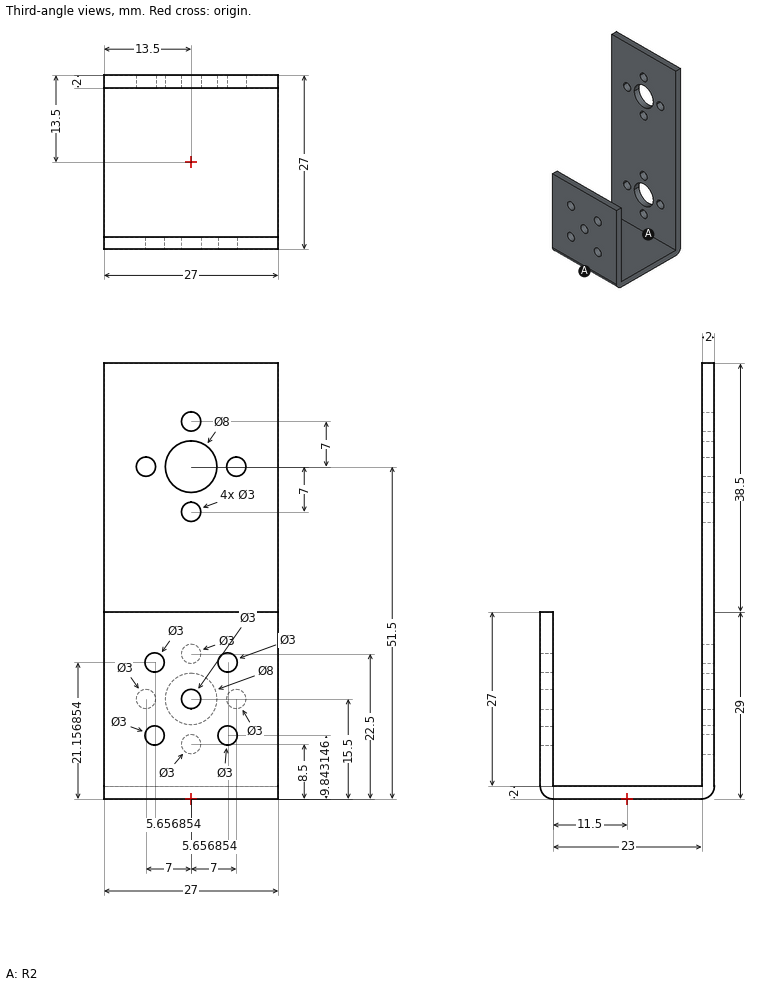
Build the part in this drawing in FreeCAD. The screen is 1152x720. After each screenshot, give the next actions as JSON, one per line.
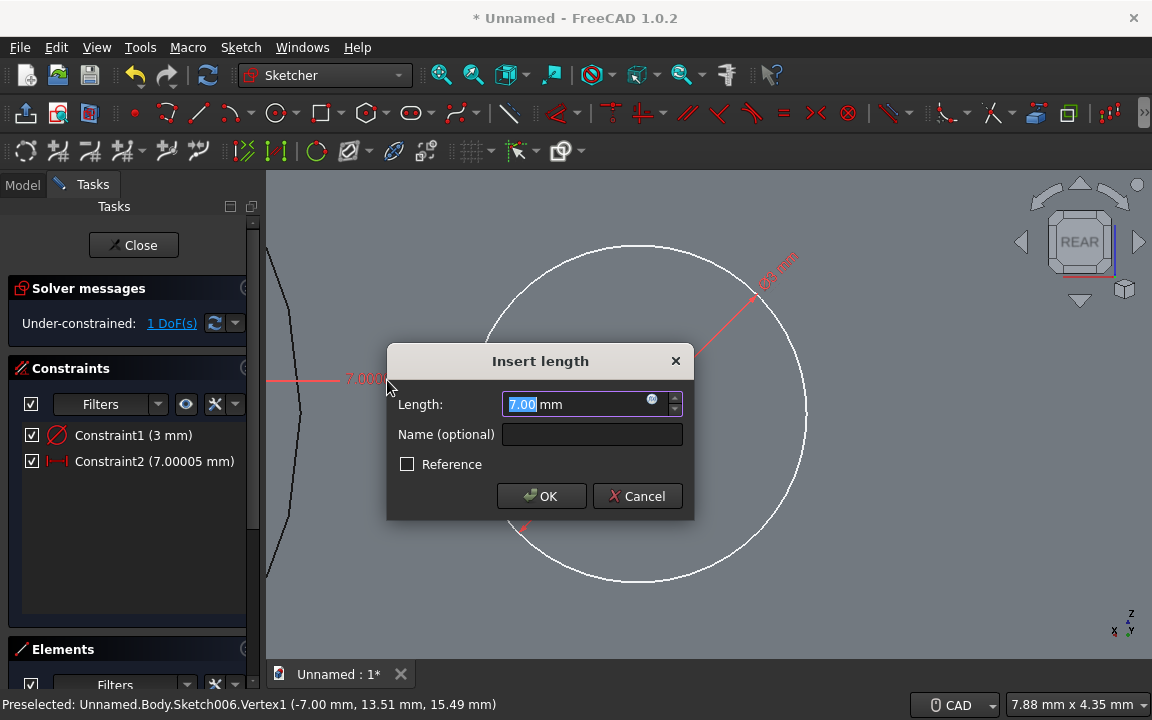
{"action": "type", "text": "7"}
{"action": "key", "text": "Return"}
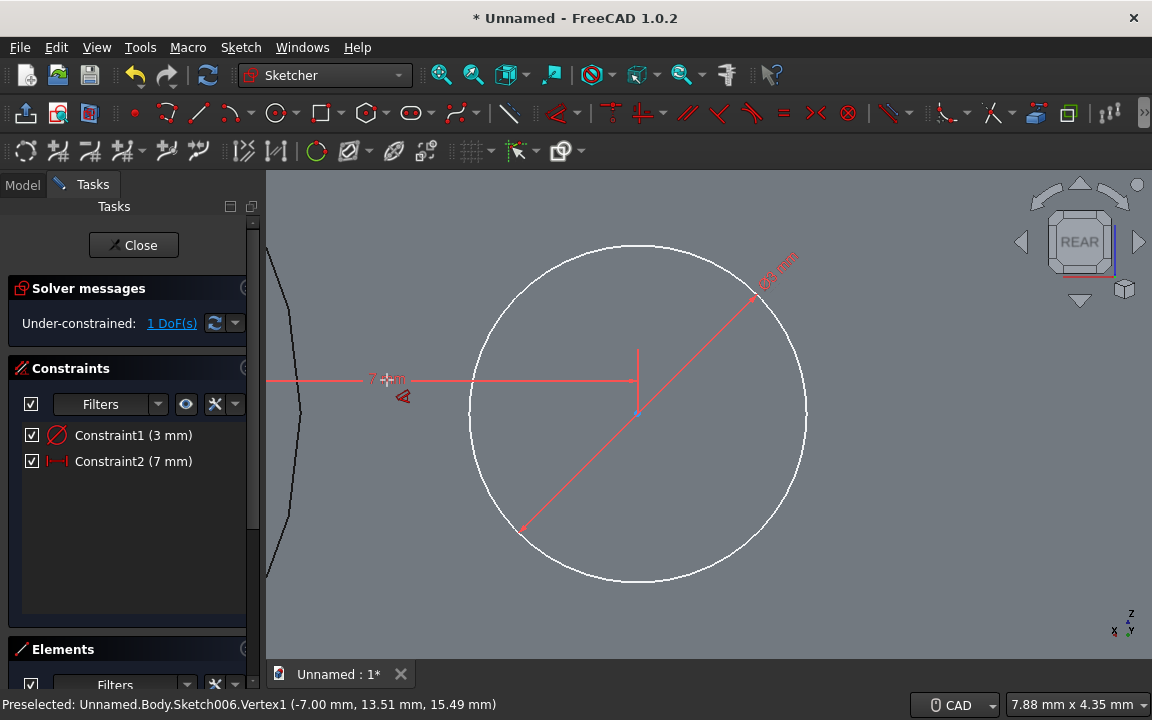
{"action": "left_click", "coordinate": [638, 414]}
{"action": "left_click", "coordinate": [672, 522]}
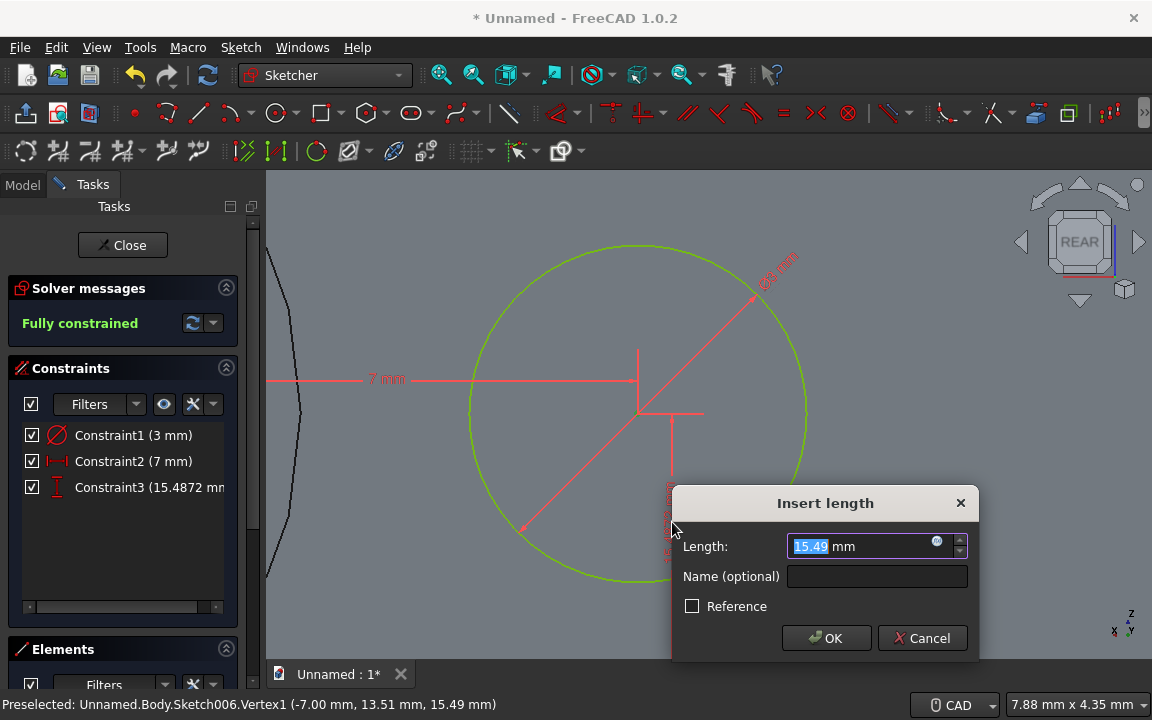
{"action": "type", "text": "15.5"}
{"action": "key", "text": "Return"}
{"action": "key", "text": "Escape"}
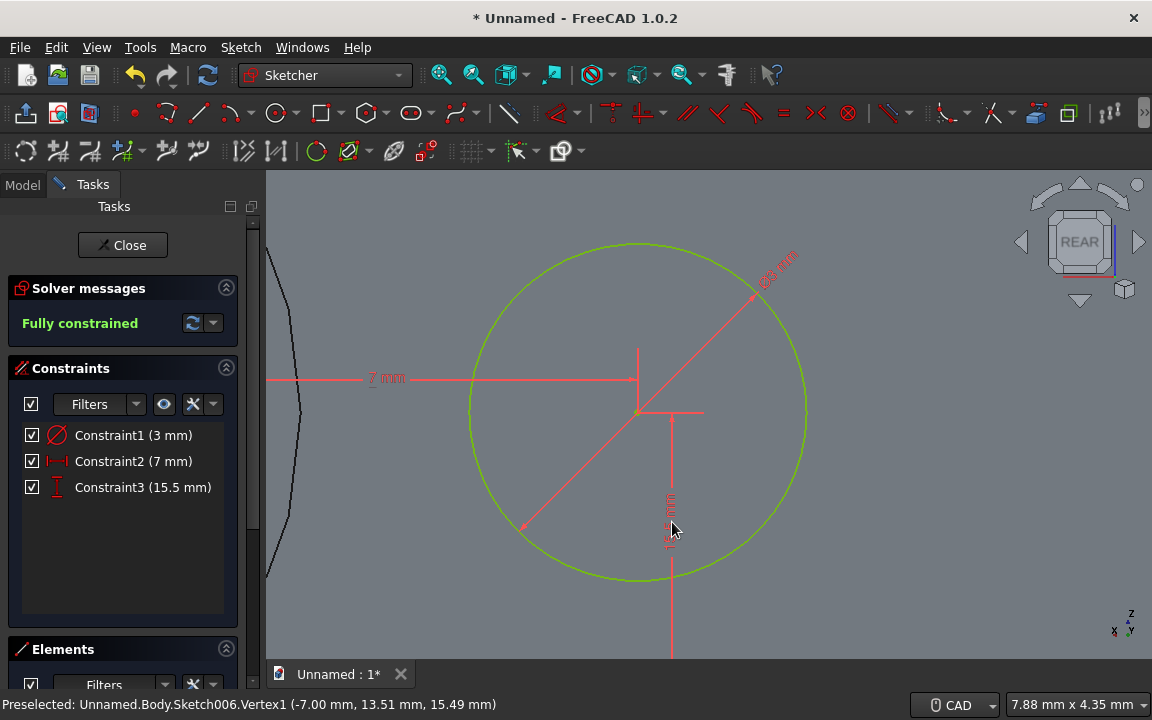
{"action": "left_click", "coordinate": [123, 245]}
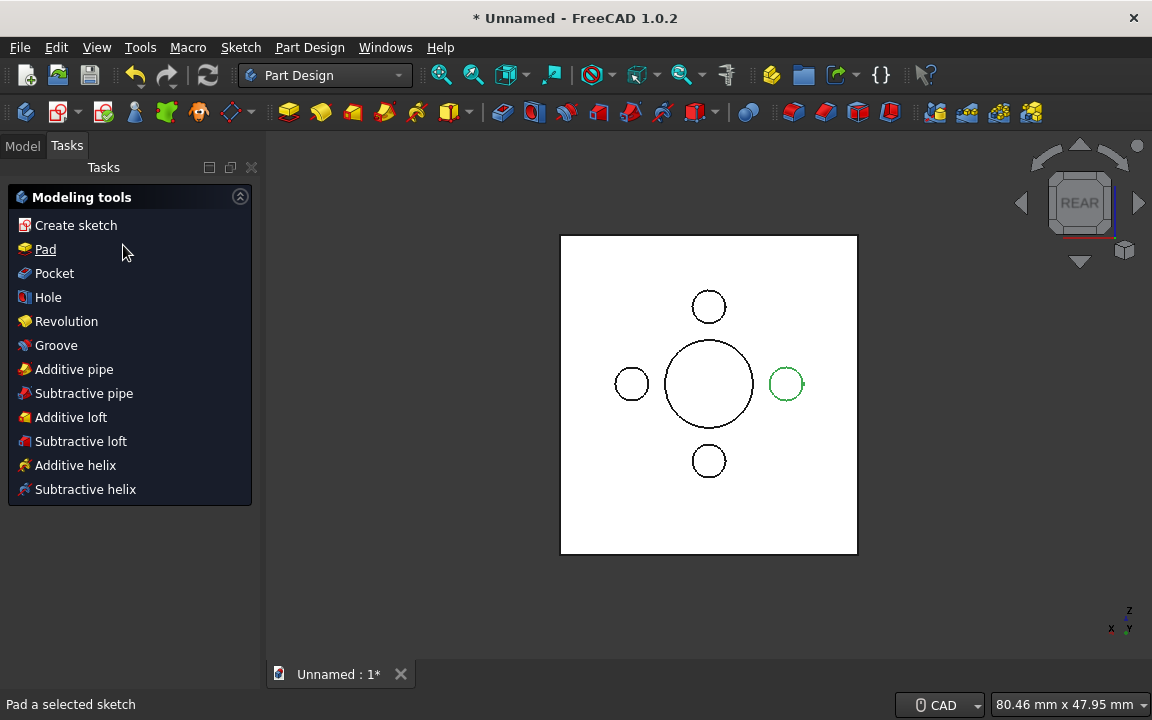
{"action": "left_click", "coordinate": [504, 112]}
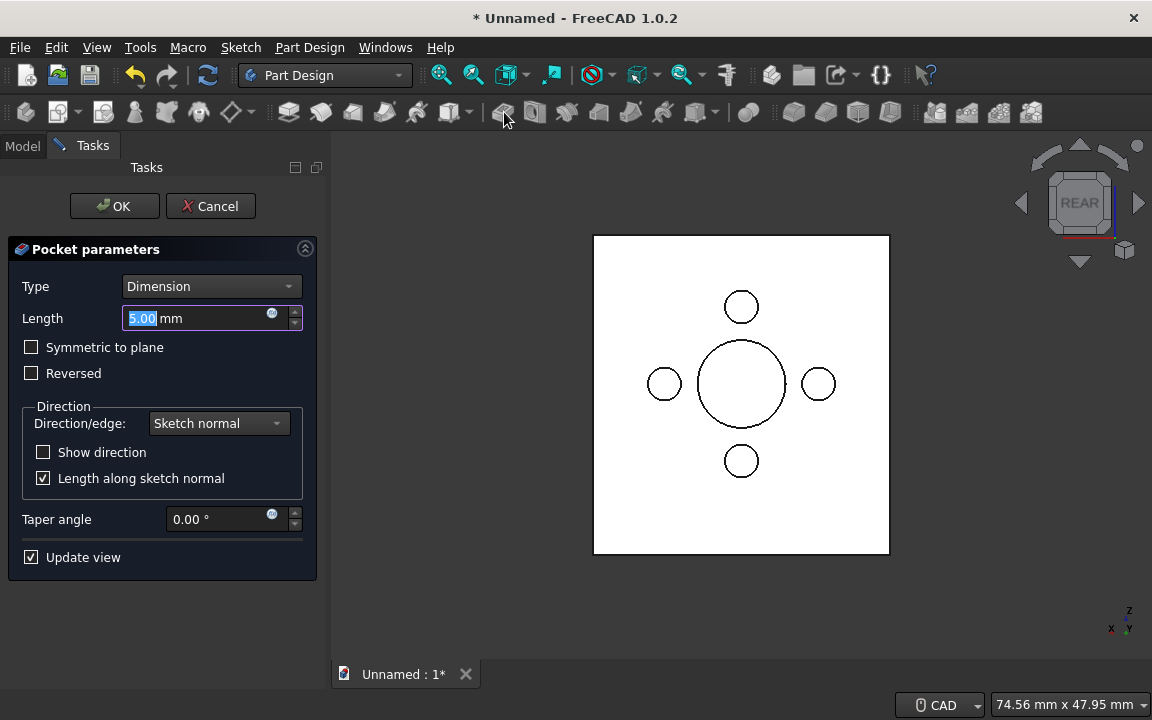
{"action": "left_click", "coordinate": [212, 286]}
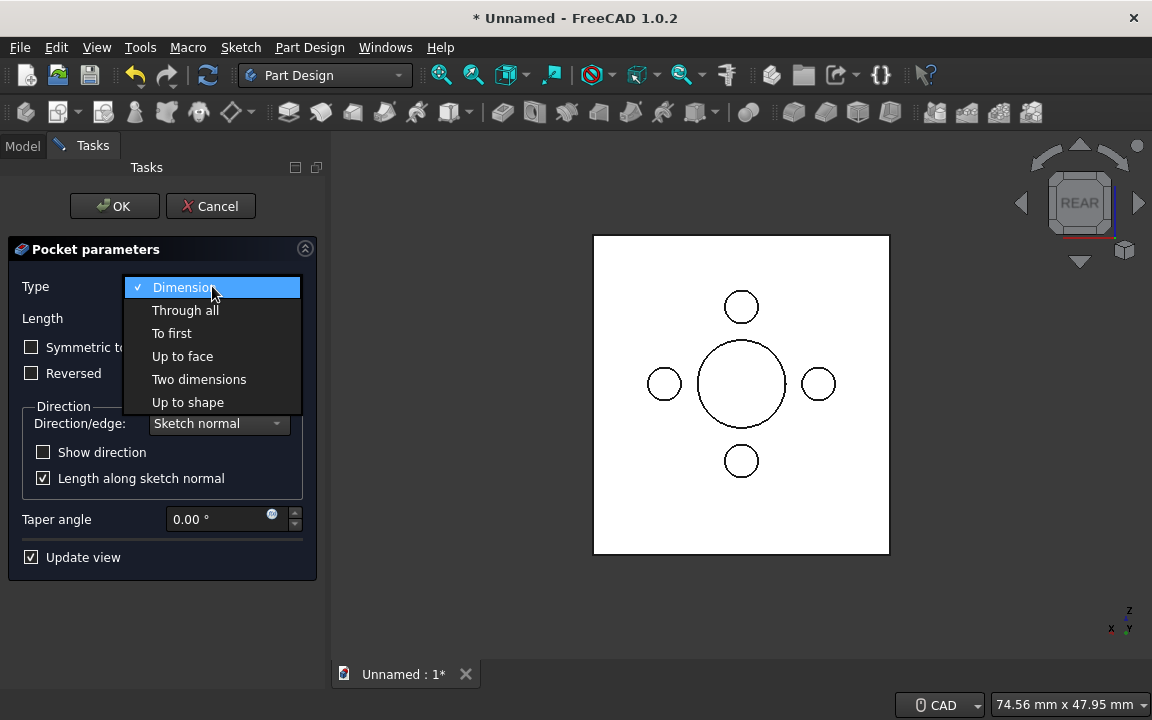
{"action": "left_click", "coordinate": [212, 334]}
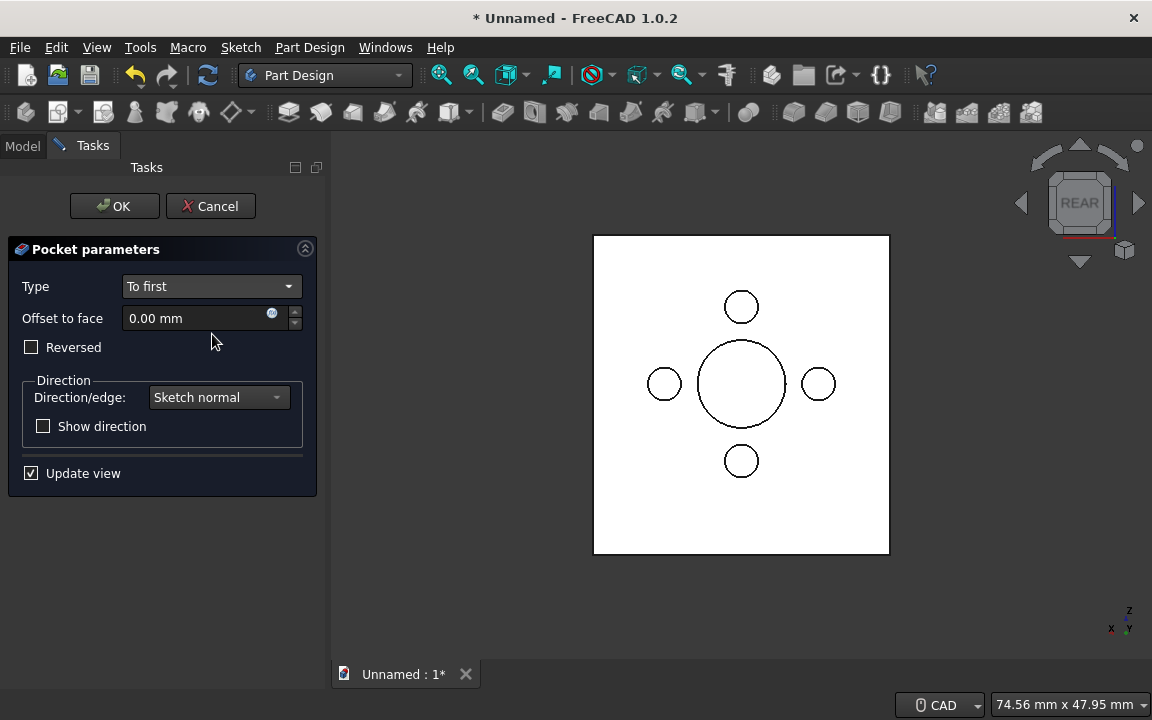
{"action": "left_click", "coordinate": [115, 206]}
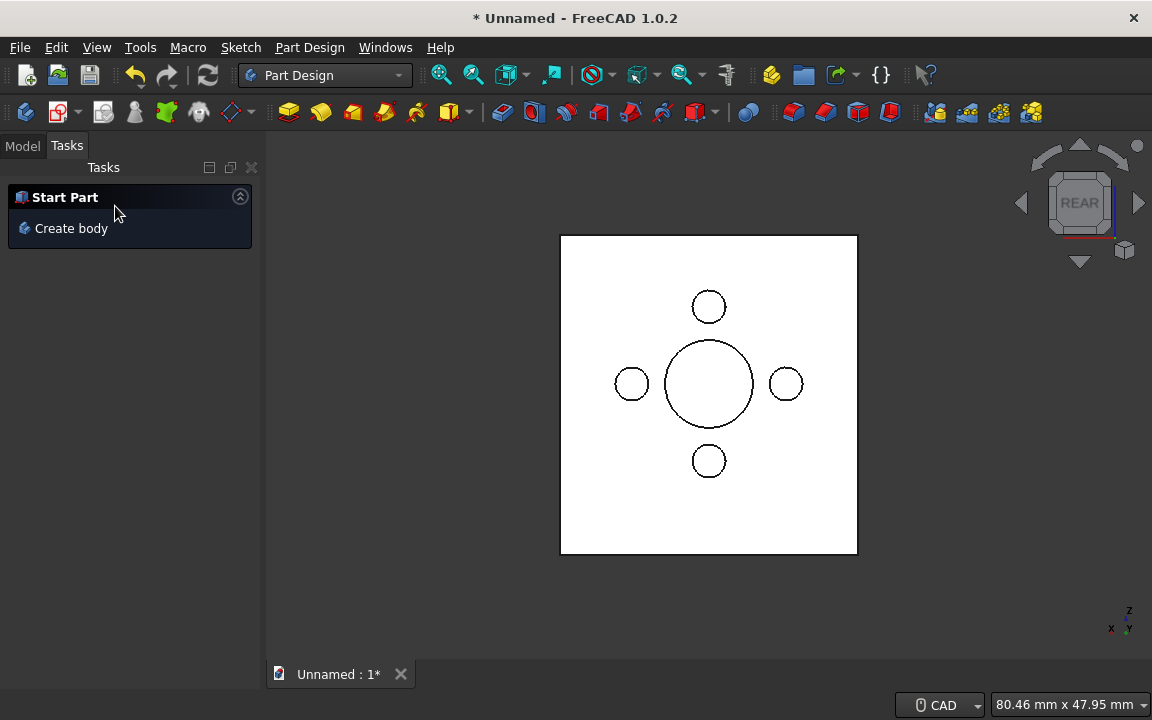
{"action": "key", "text": "0"}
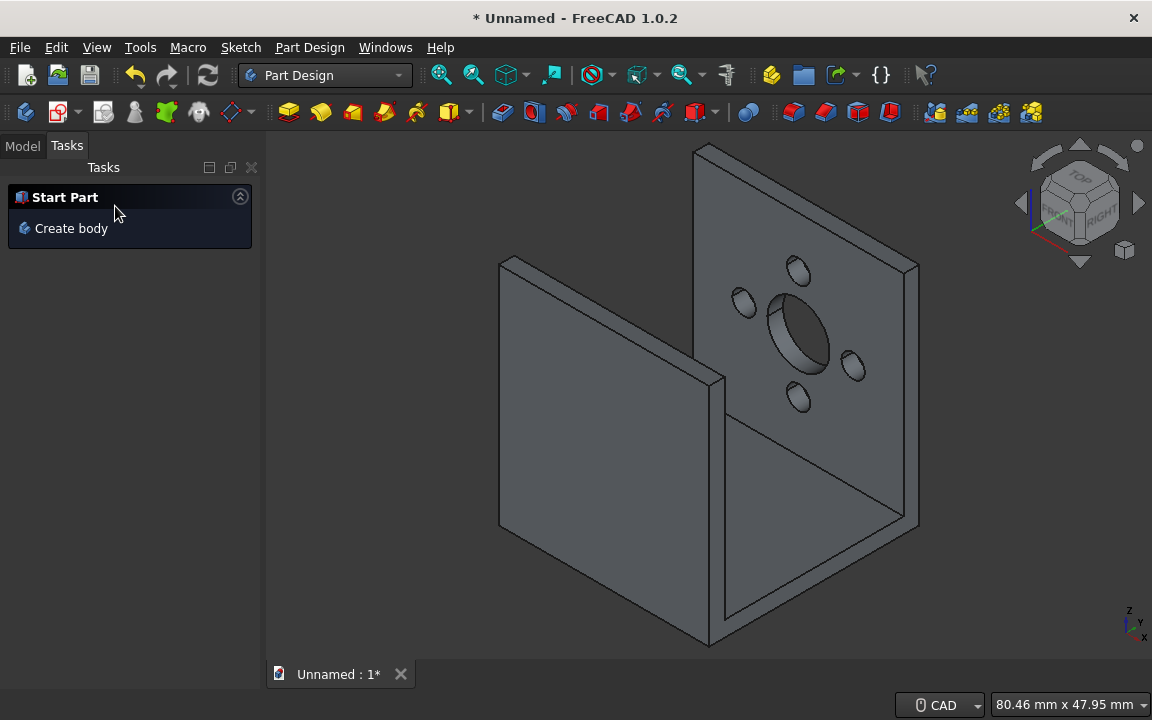
{"action": "left_click", "coordinate": [604, 455]}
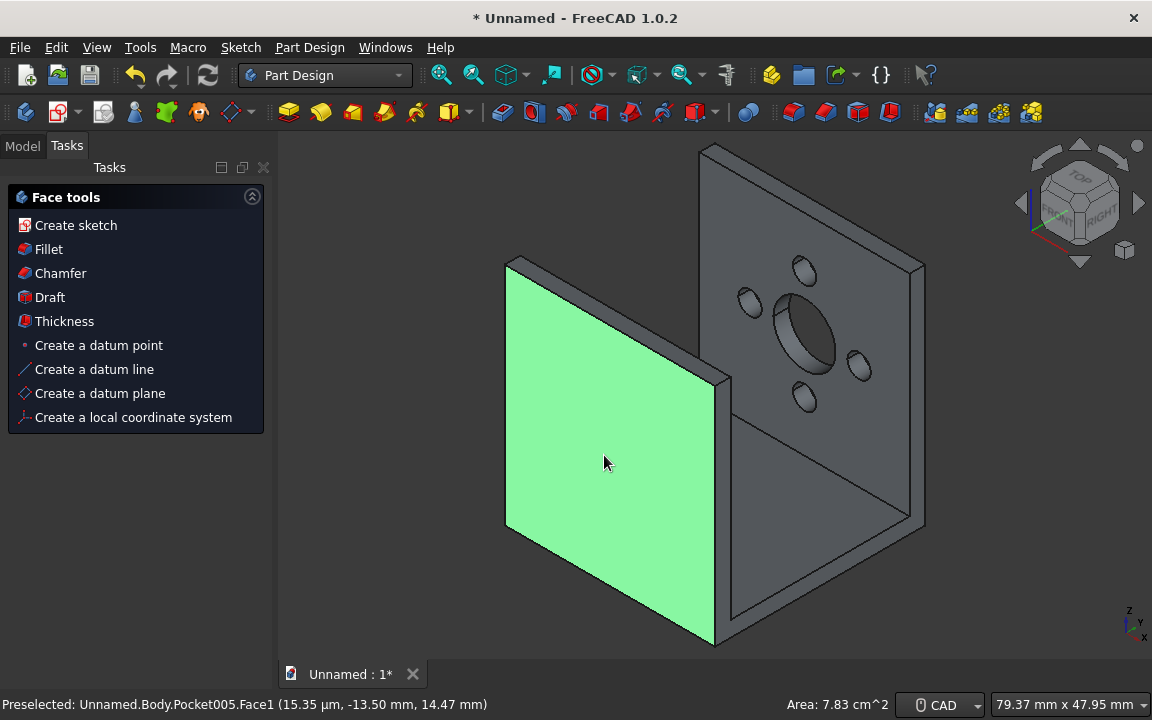
{"action": "left_click", "coordinate": [58, 112]}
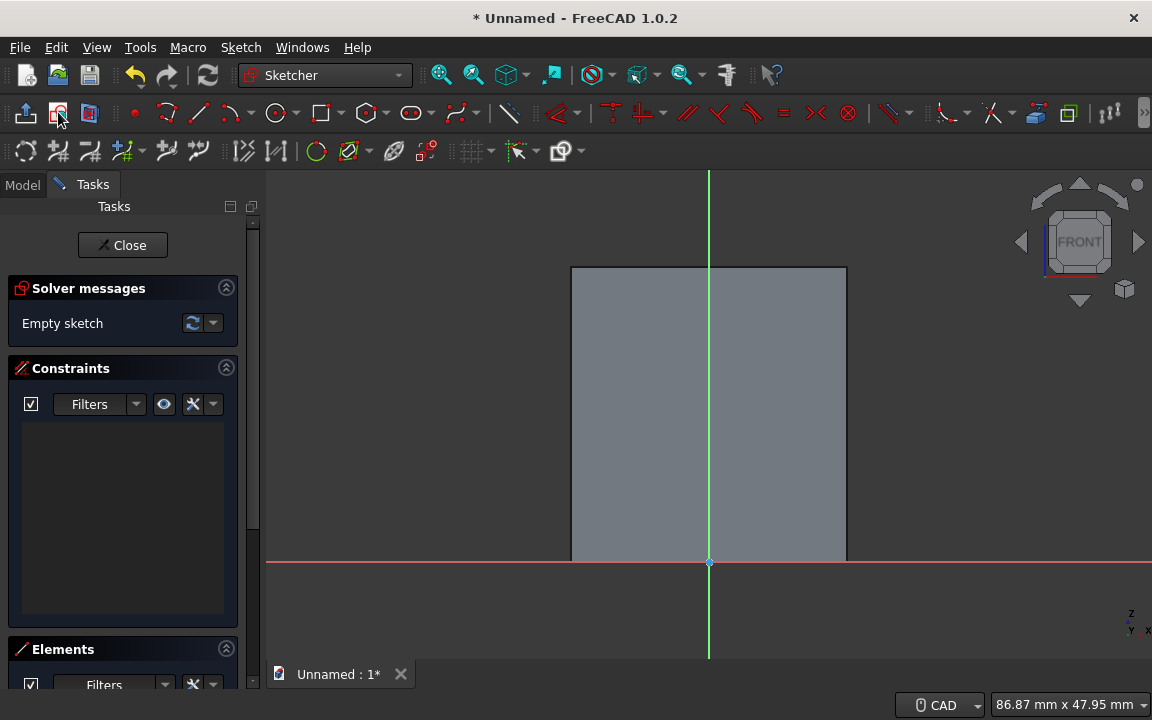
{"action": "scroll", "coordinate": [716, 403], "scroll_direction": "up", "scroll_amount": 12}